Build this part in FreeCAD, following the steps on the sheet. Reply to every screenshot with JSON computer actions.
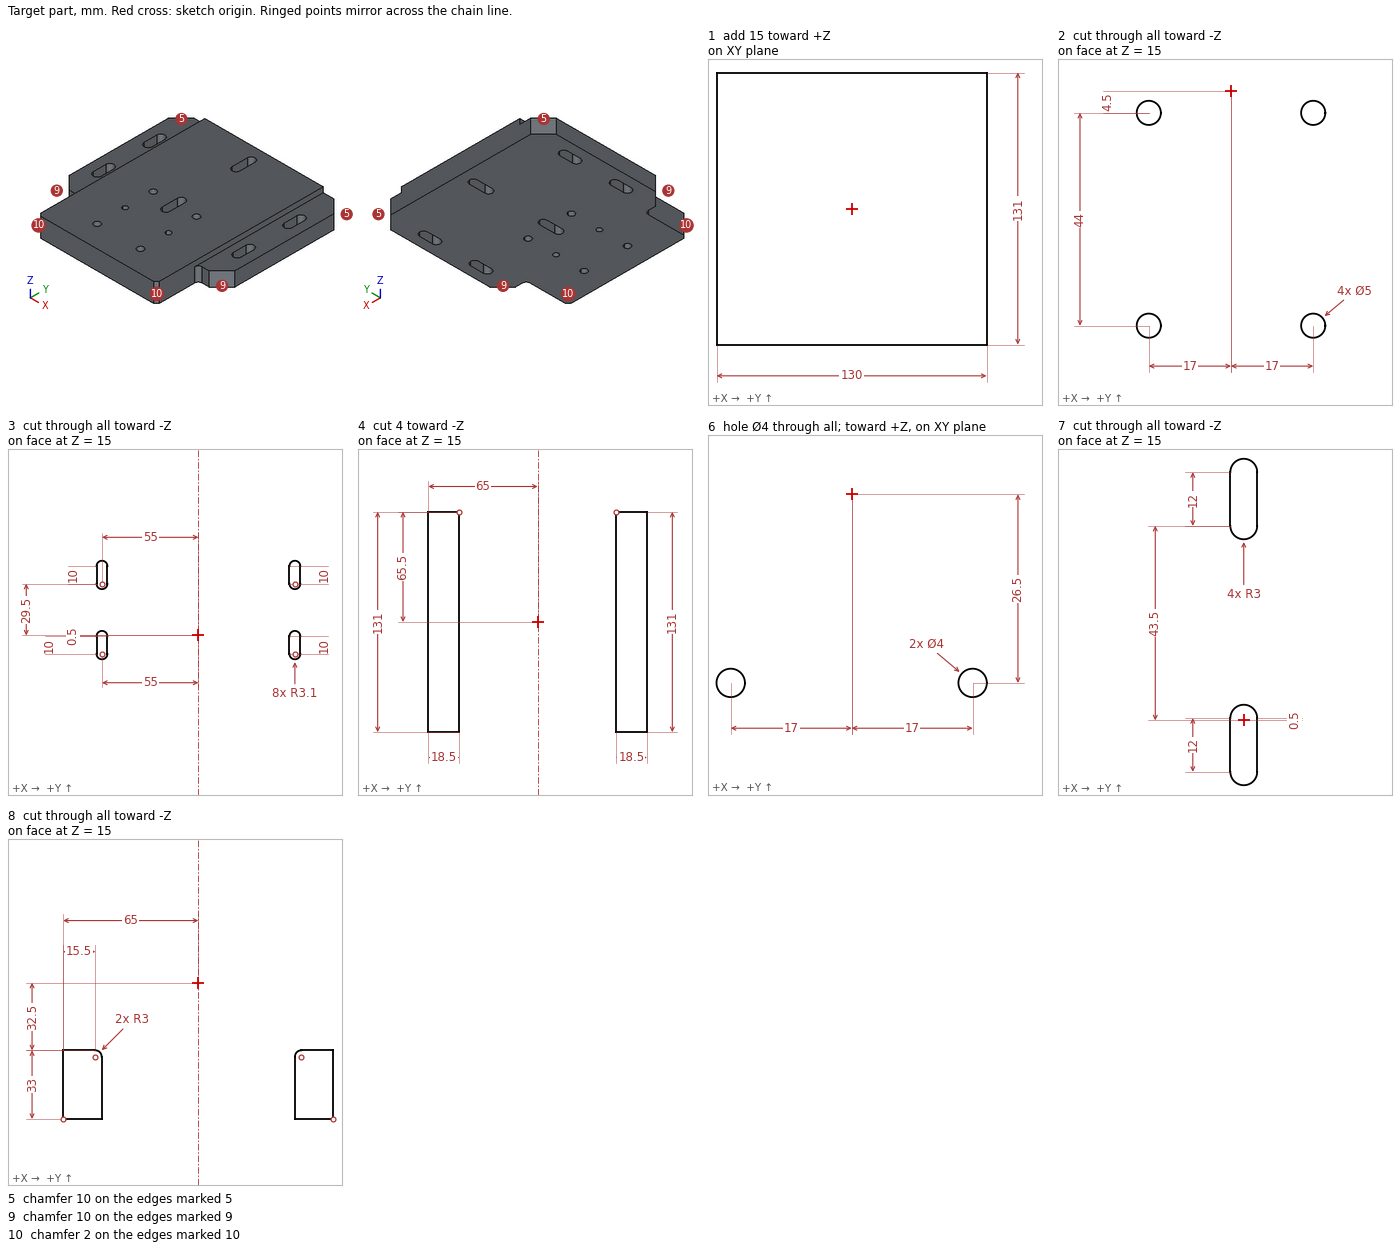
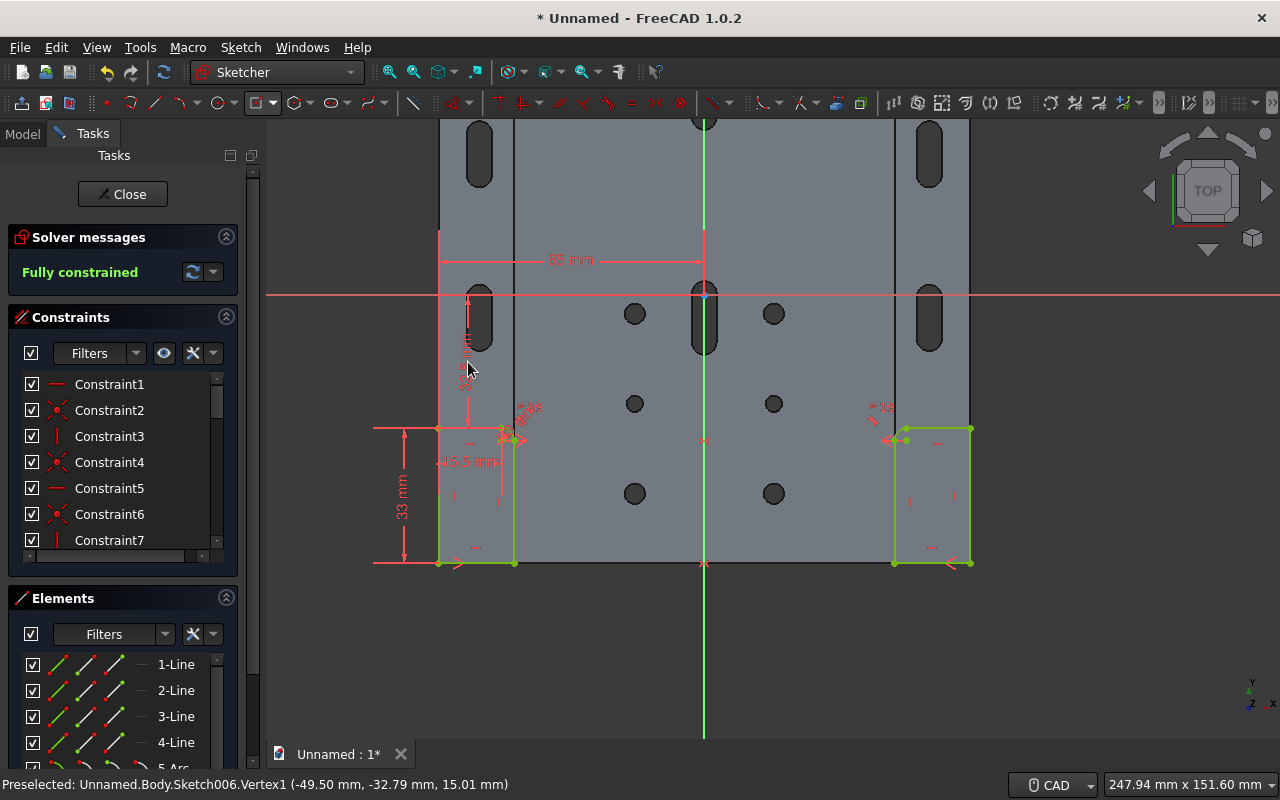
{"action": "left_click", "coordinate": [123, 194]}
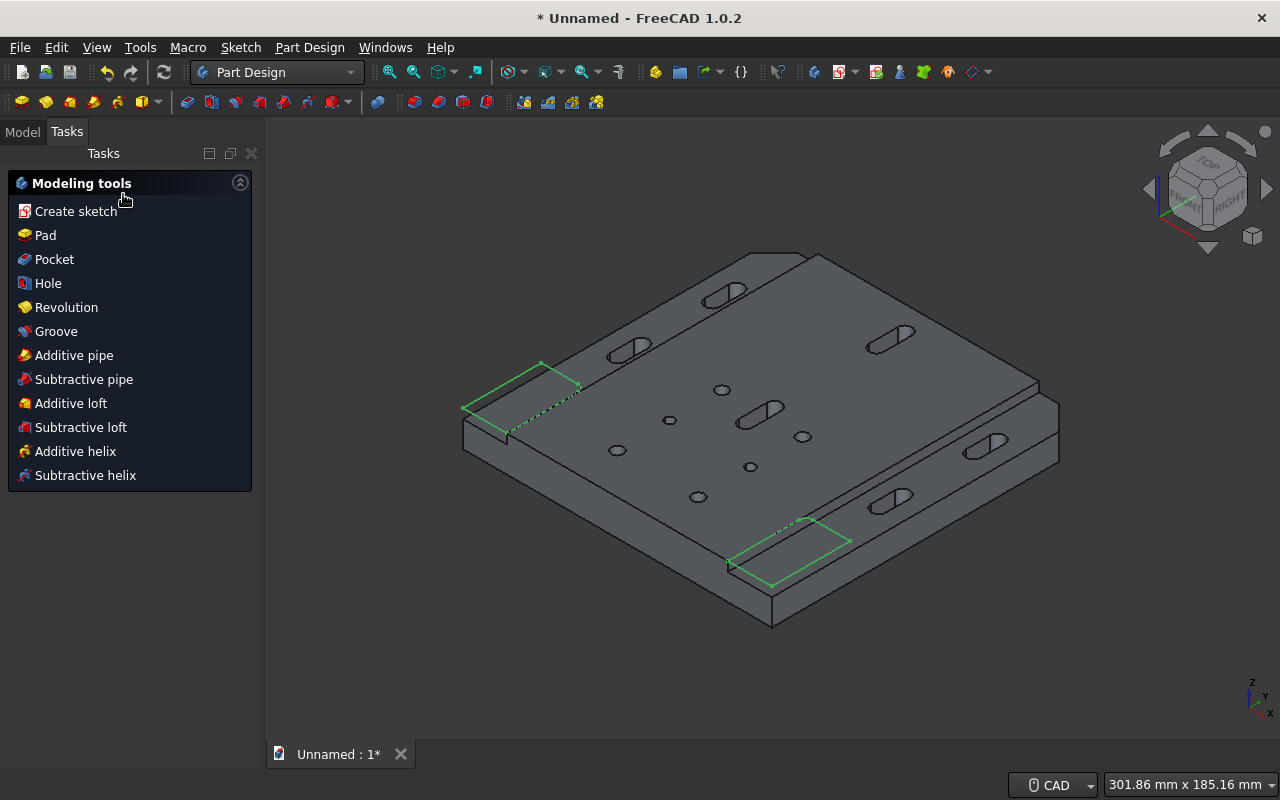
{"action": "left_click", "coordinate": [188, 102]}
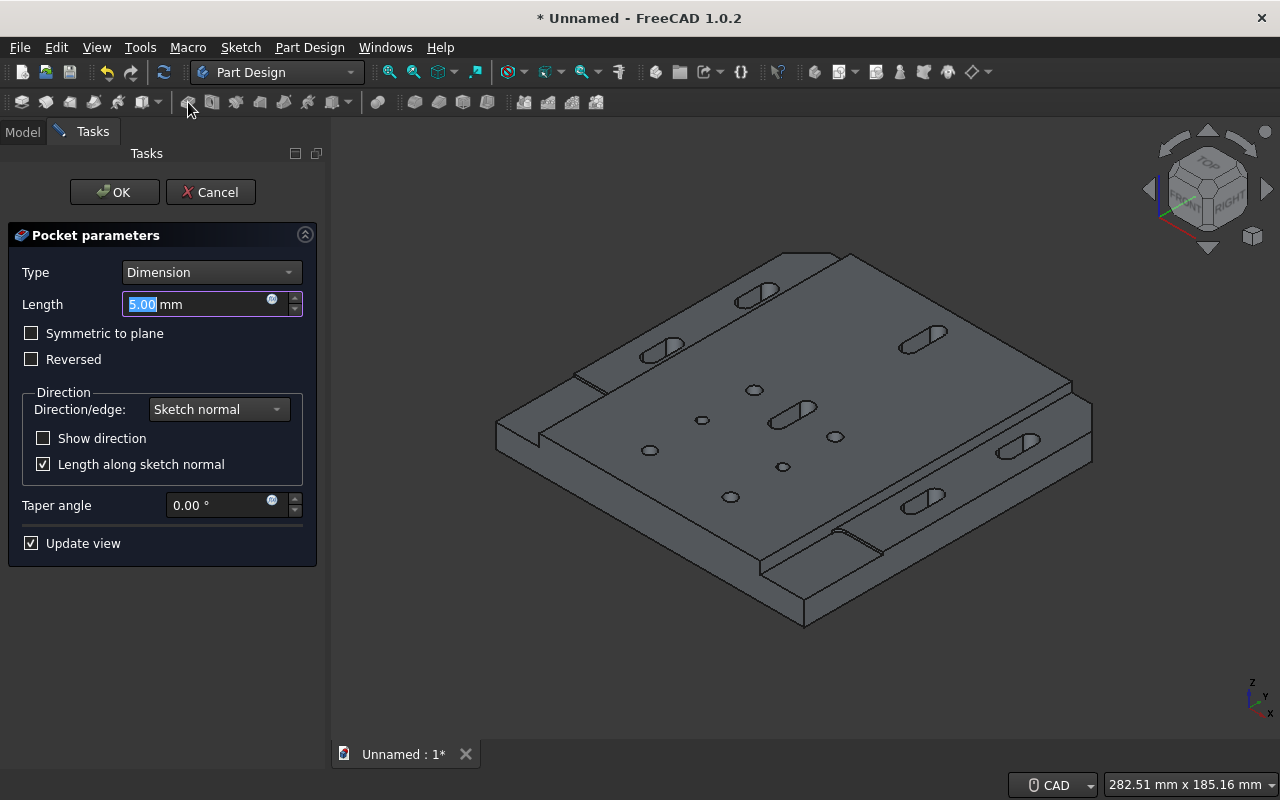
{"action": "left_click", "coordinate": [212, 272]}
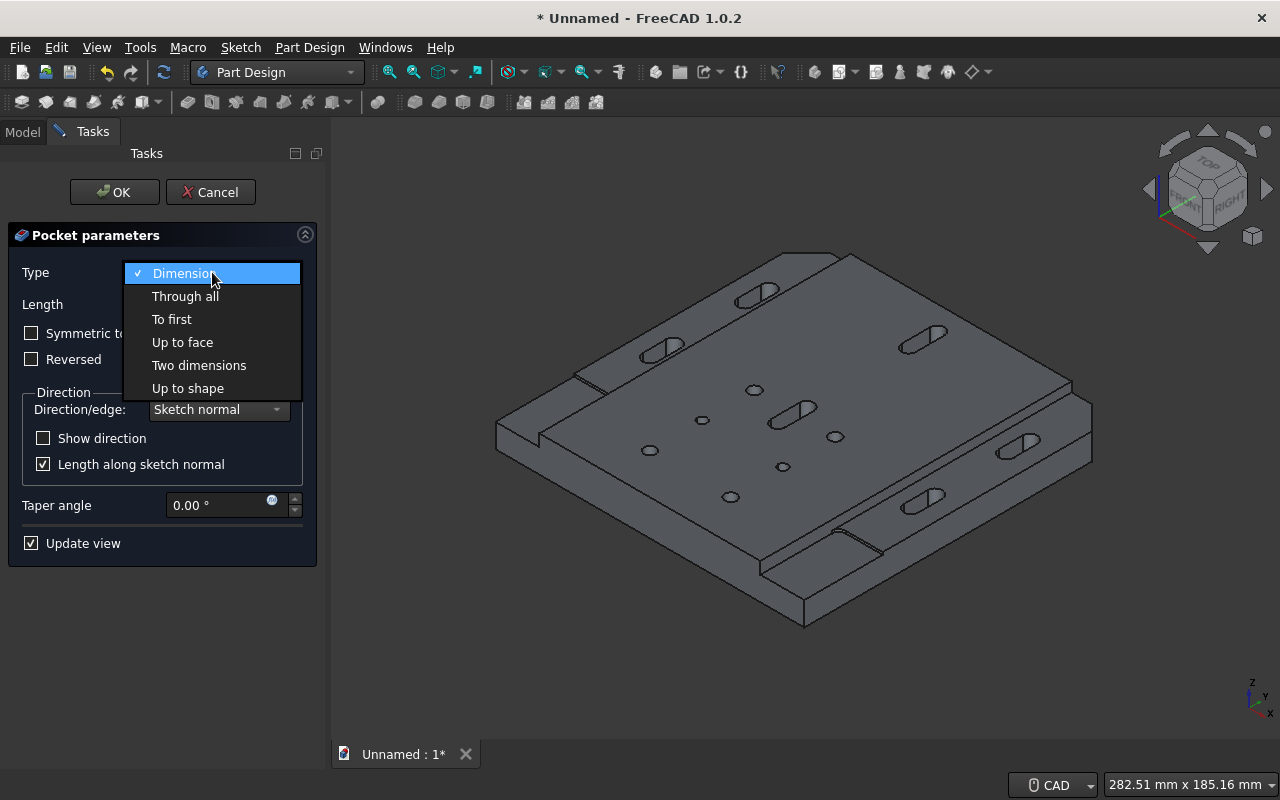
{"action": "left_click", "coordinate": [212, 296]}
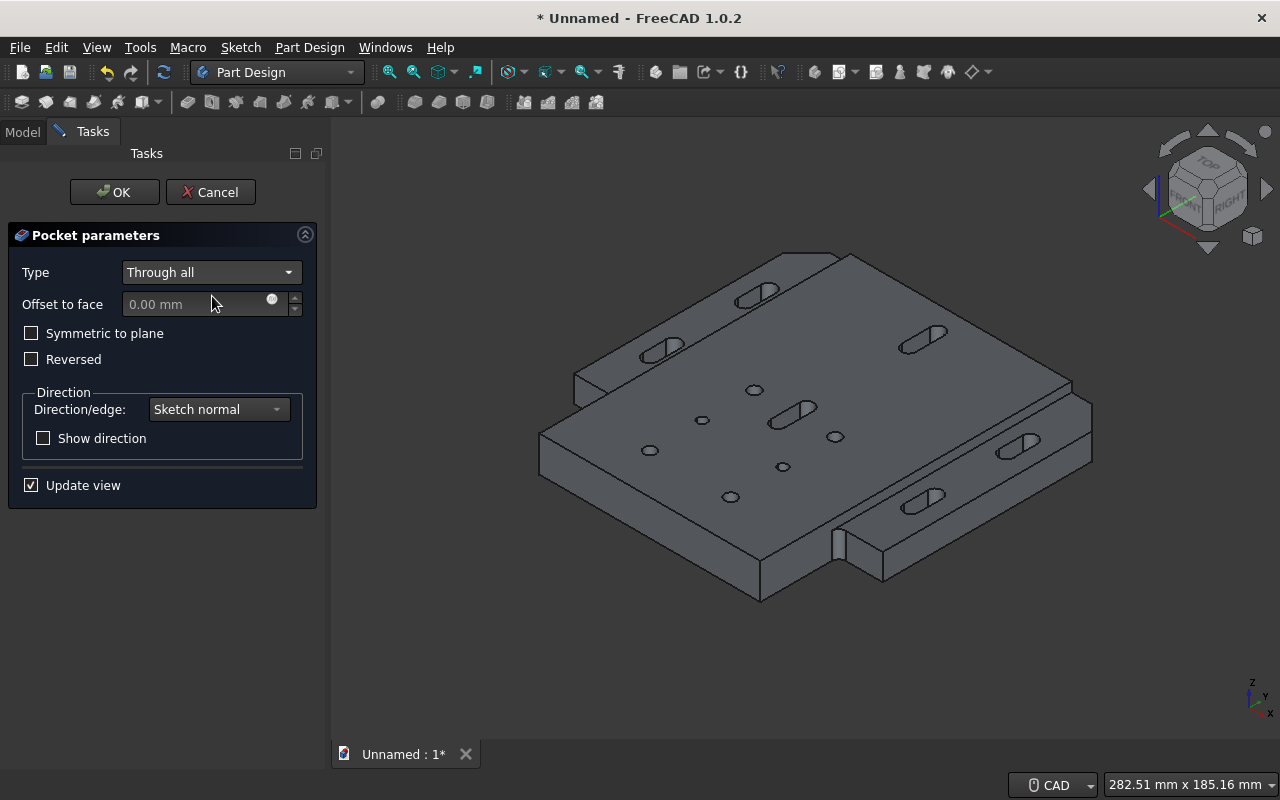
{"action": "left_click", "coordinate": [115, 192]}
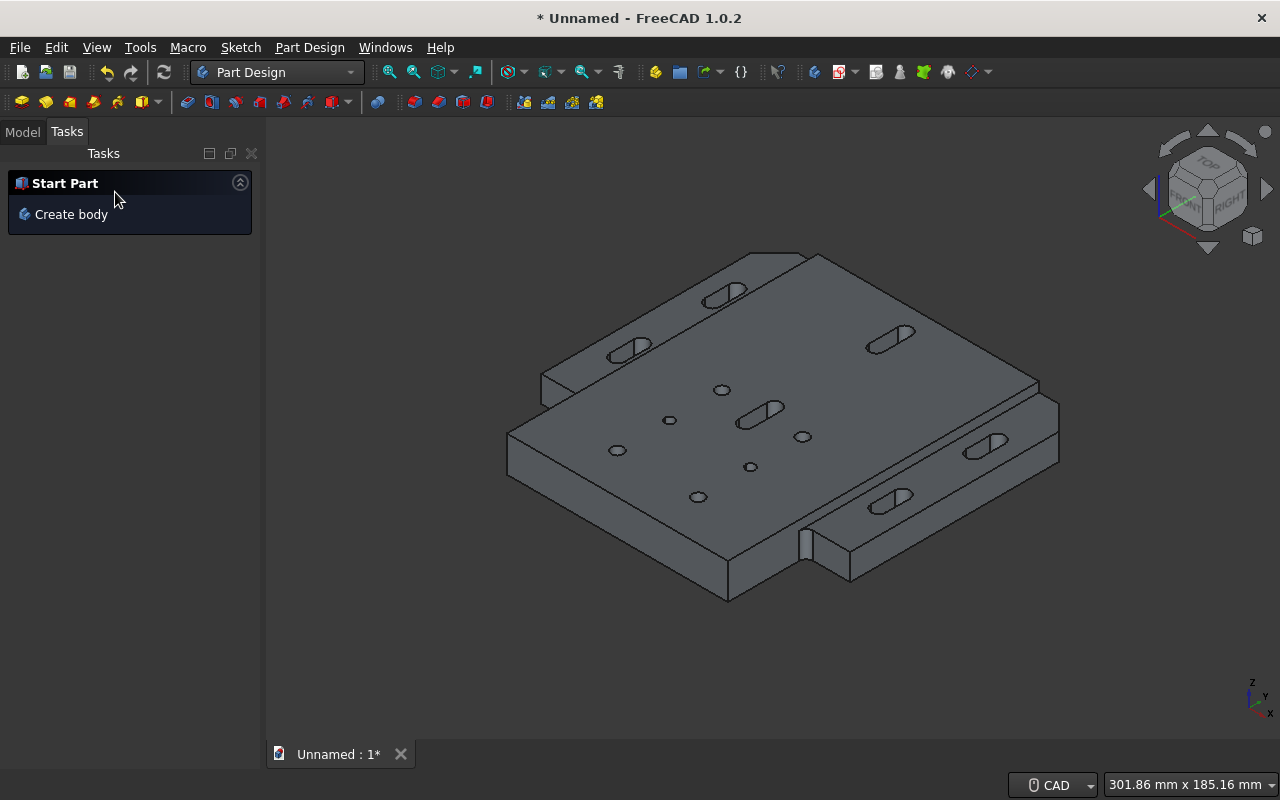
{"action": "left_click", "coordinate": [850, 566]}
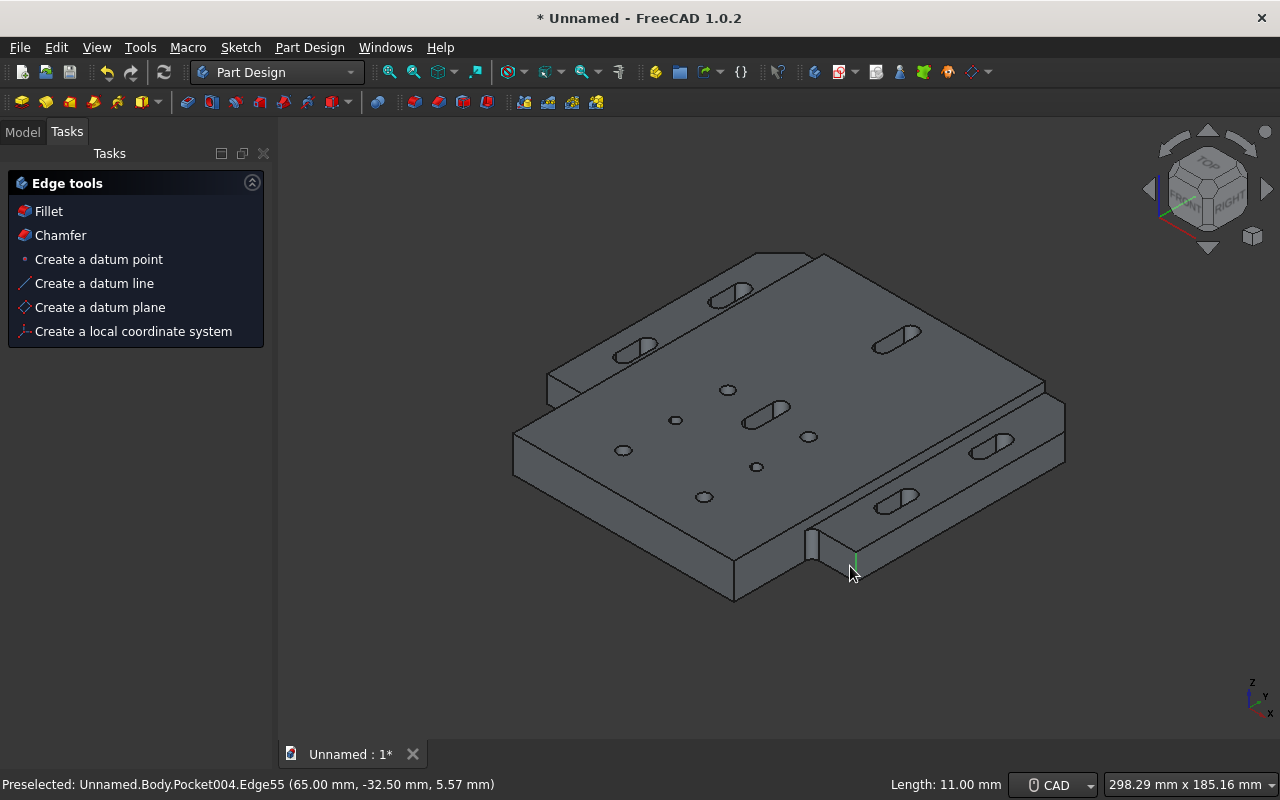
{"action": "key", "text": "2"}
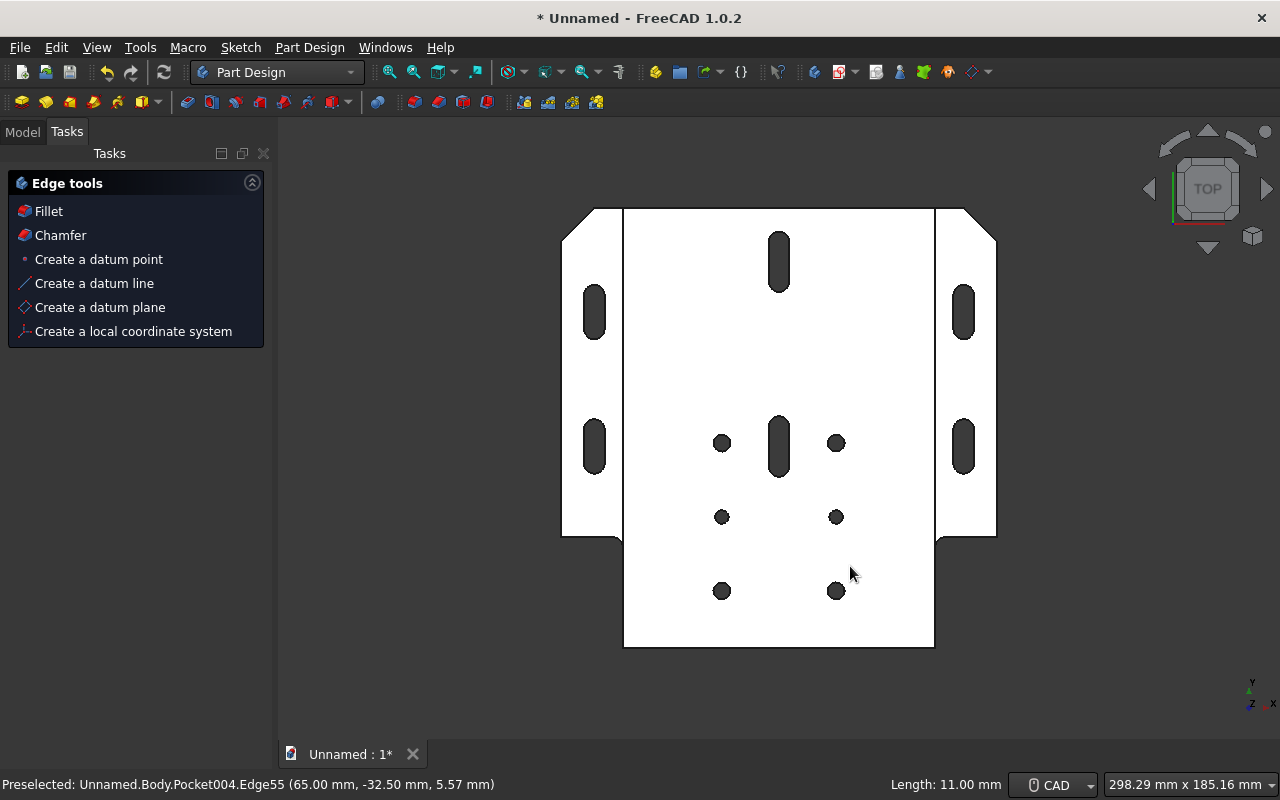
{"action": "key", "text": "0"}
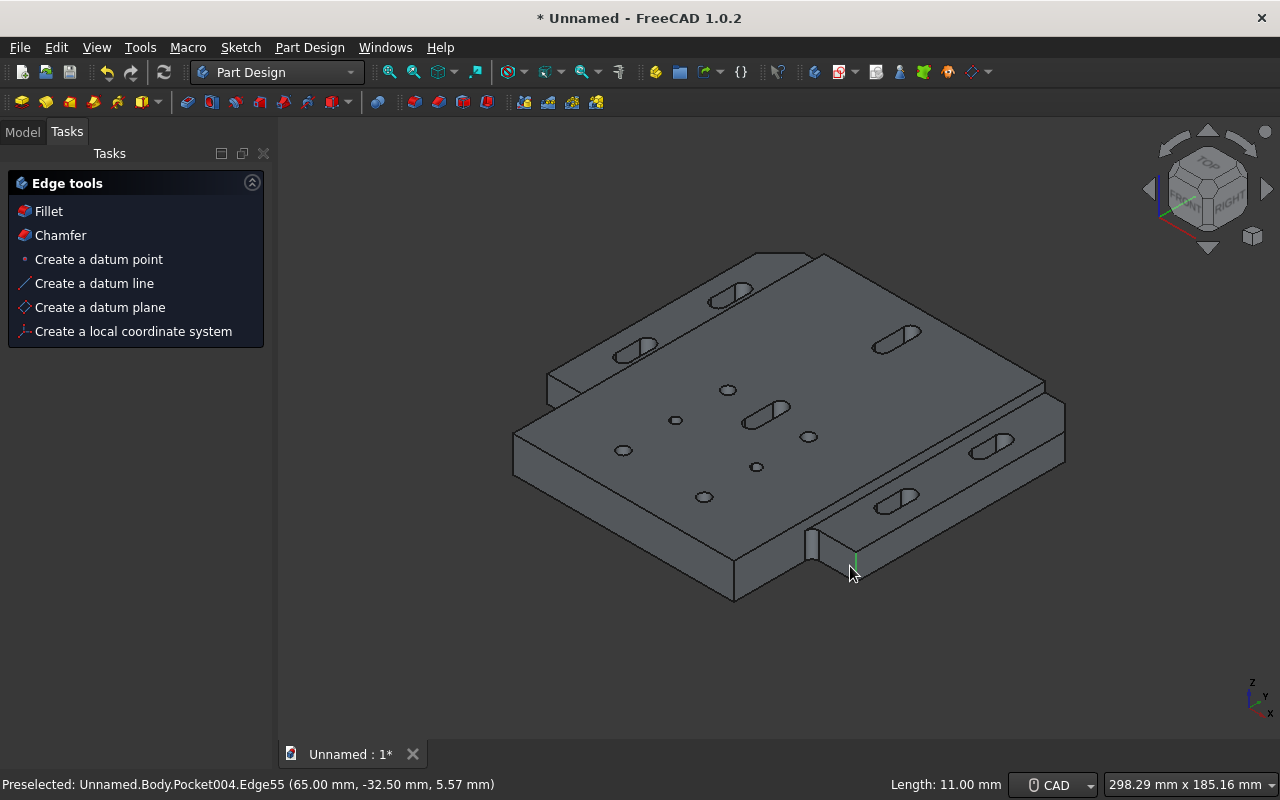
{"action": "key", "text": "1"}